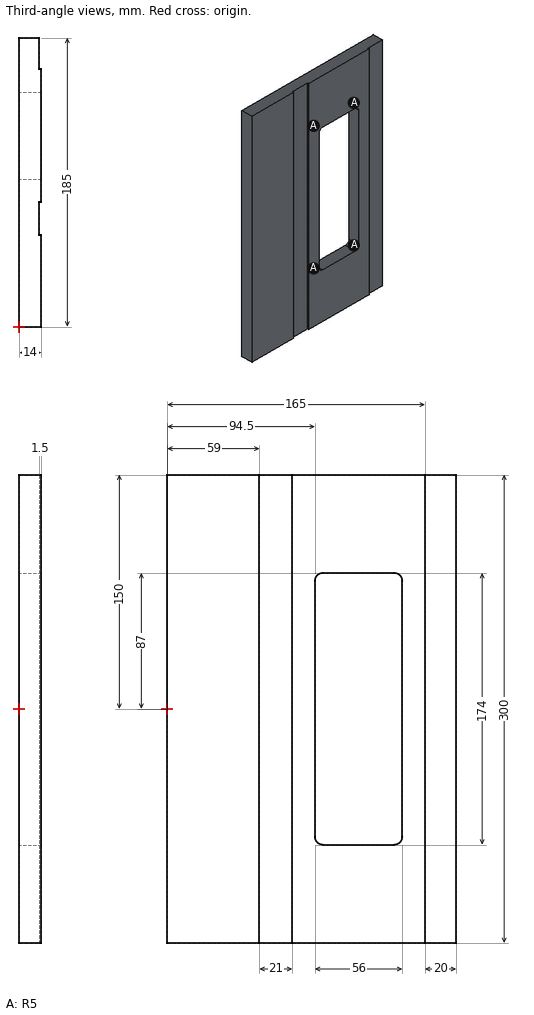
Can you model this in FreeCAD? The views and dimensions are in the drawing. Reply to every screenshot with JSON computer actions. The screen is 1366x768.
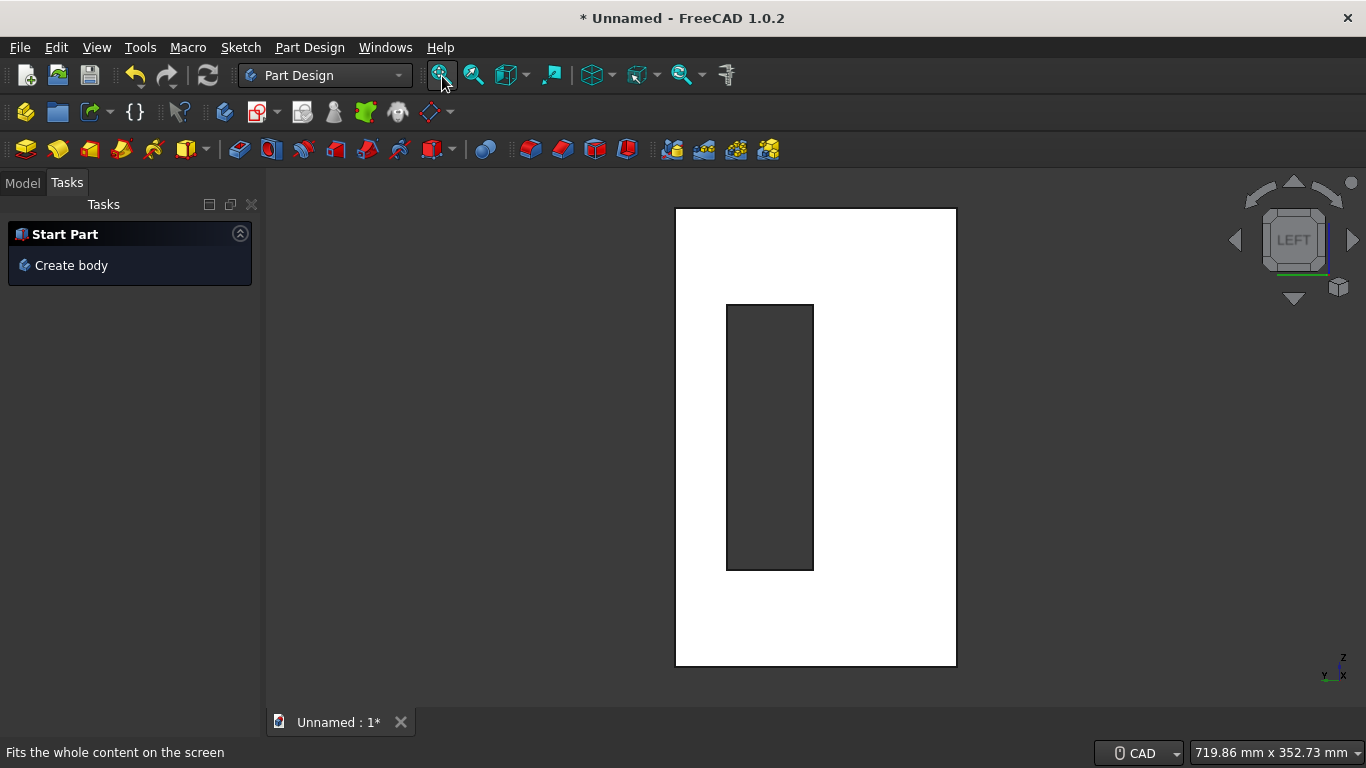
{"action": "key", "text": "0"}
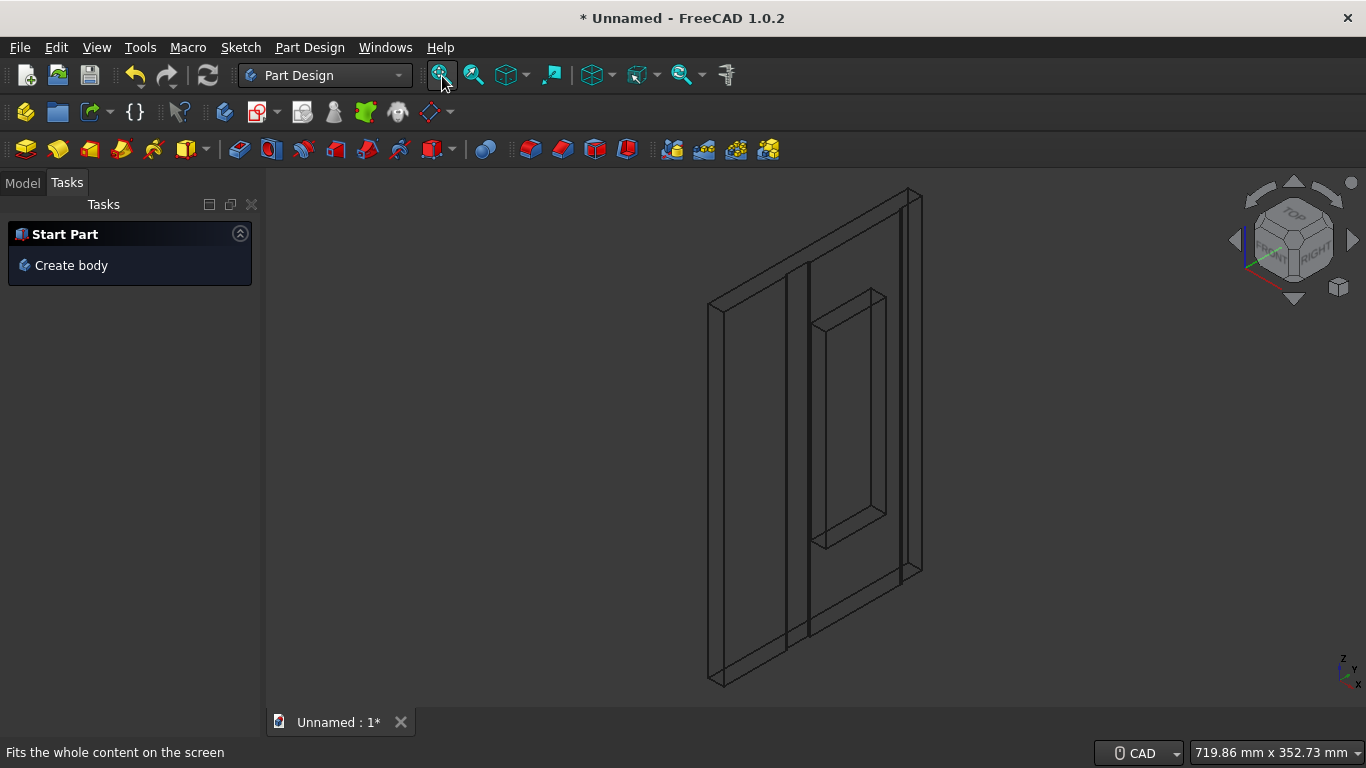
{"action": "left_click", "coordinate": [879, 509]}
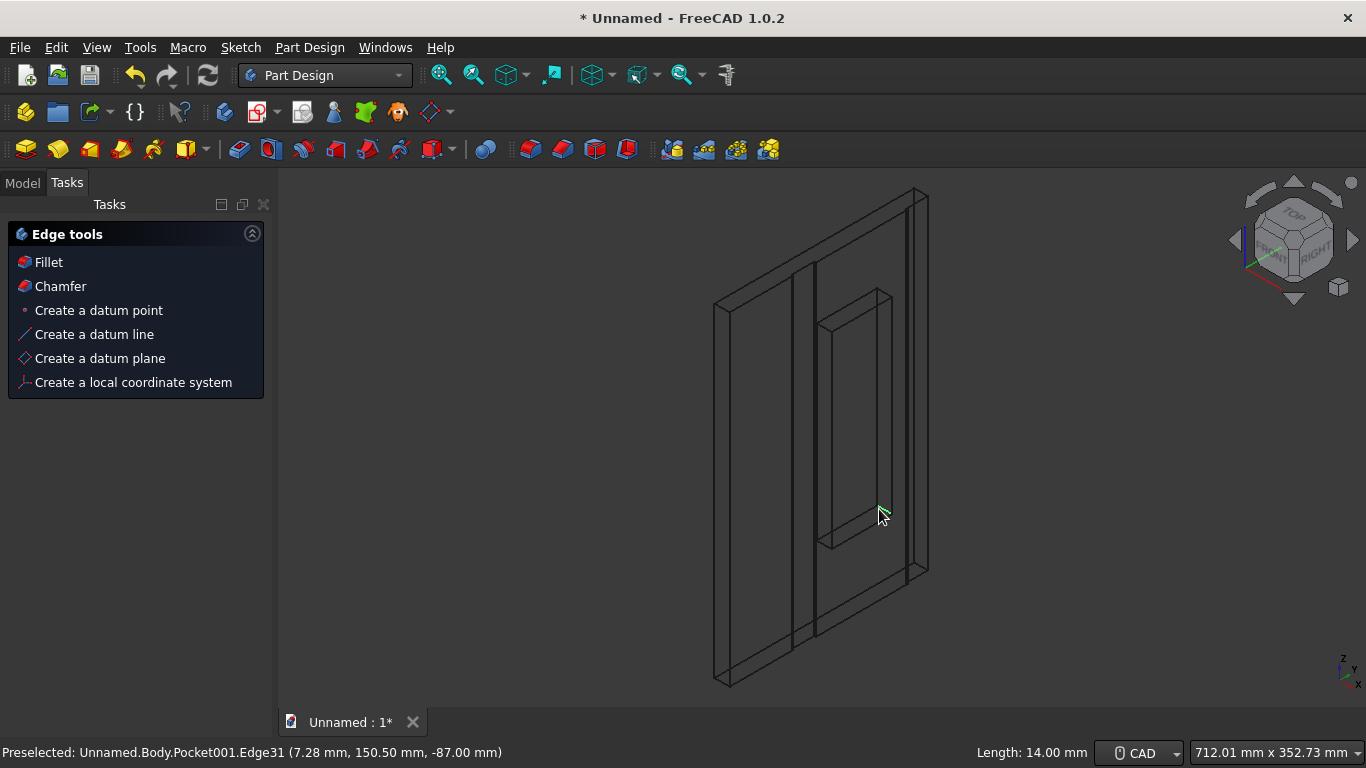
{"action": "left_click", "coordinate": [824, 544], "text": "ctrl"}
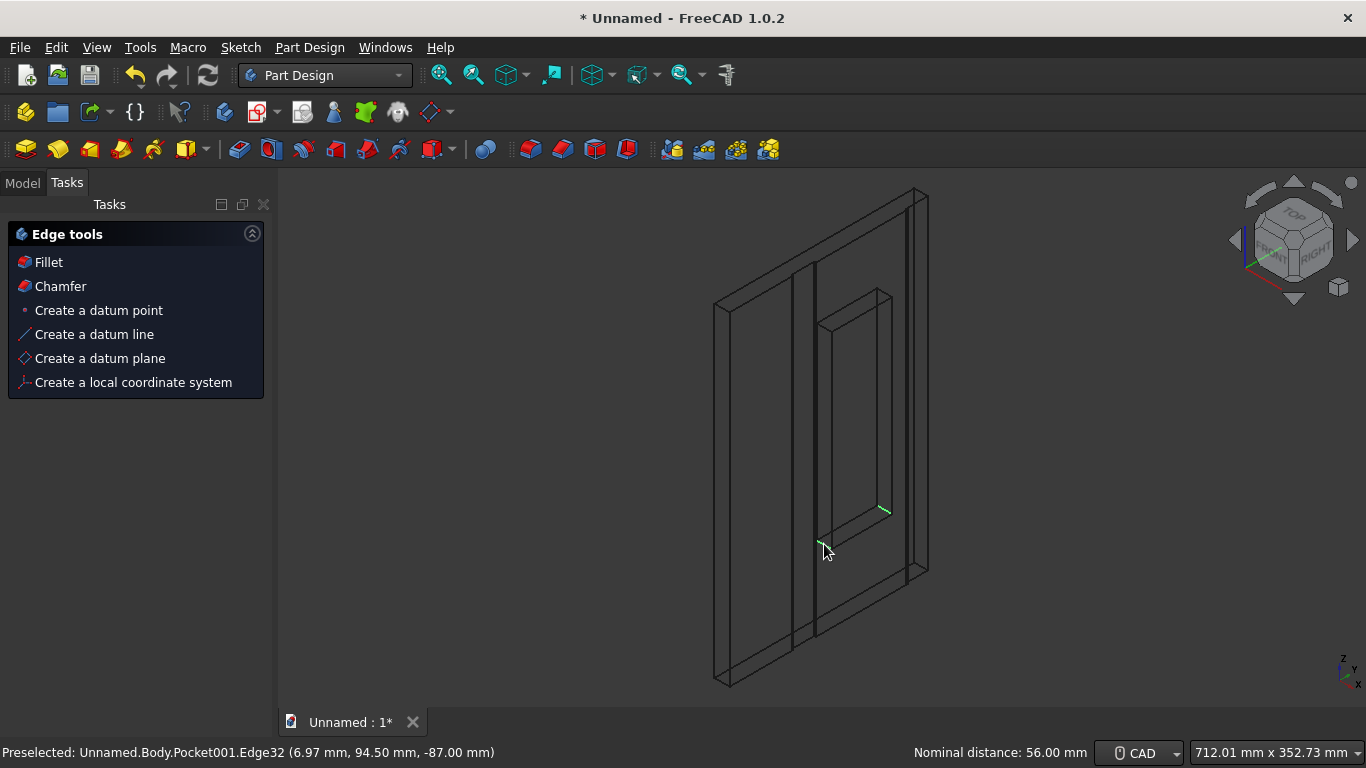
{"action": "left_click", "coordinate": [824, 327], "text": "ctrl"}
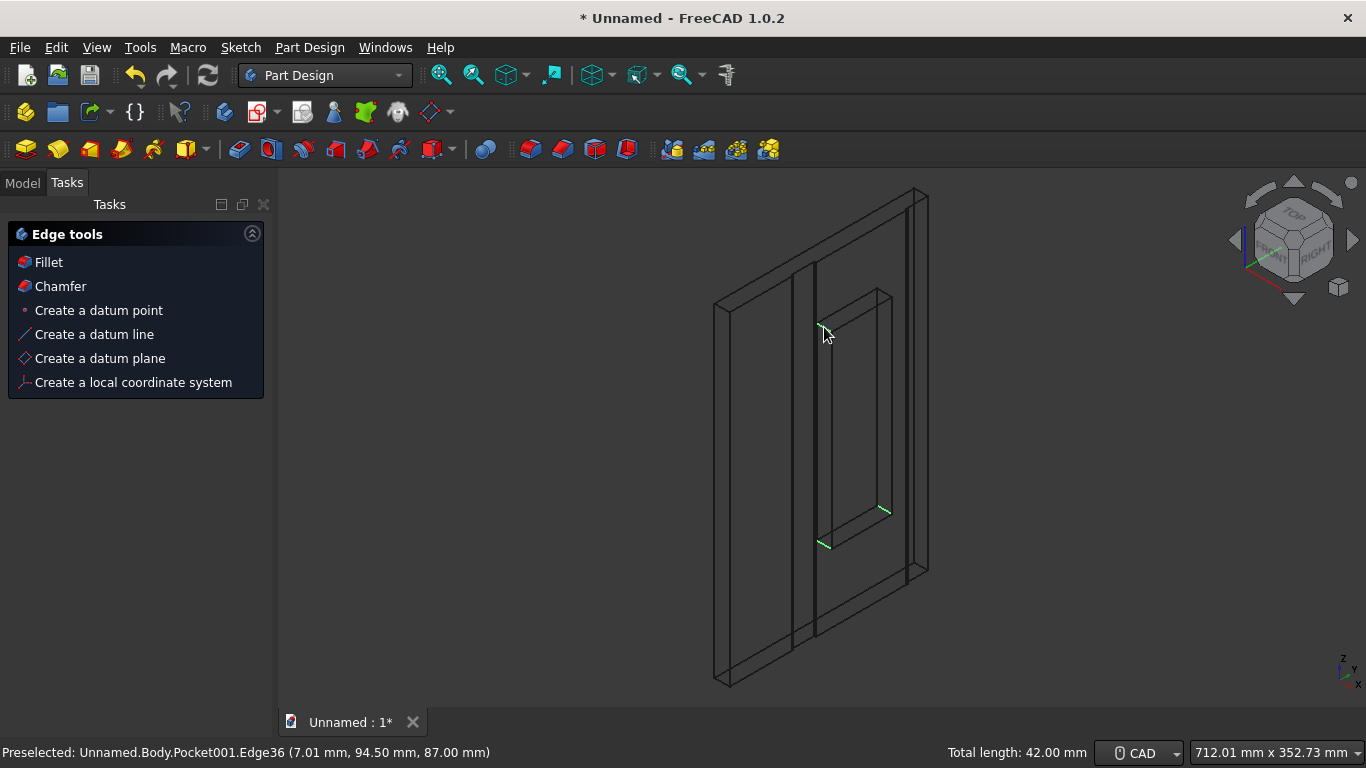
{"action": "left_click", "coordinate": [885, 292], "text": "ctrl"}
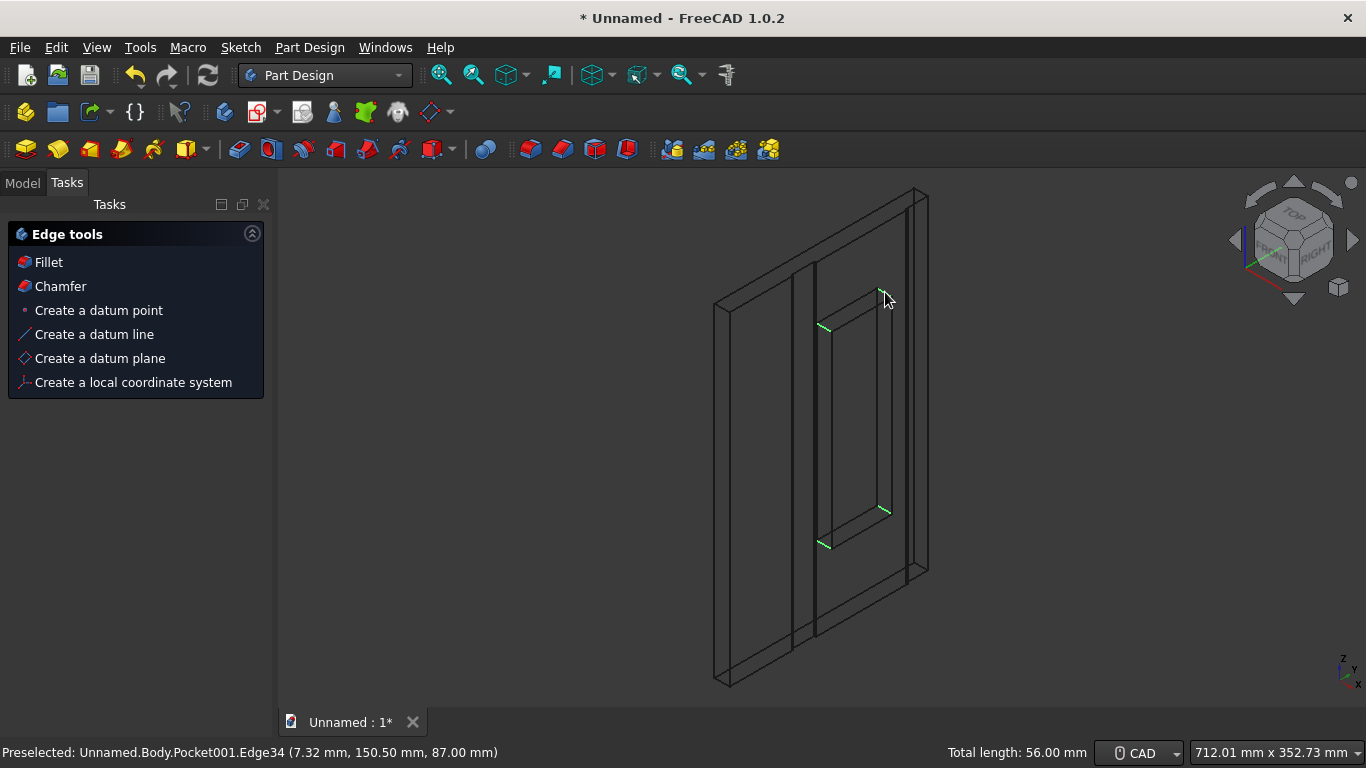
{"action": "key", "text": "v 1"}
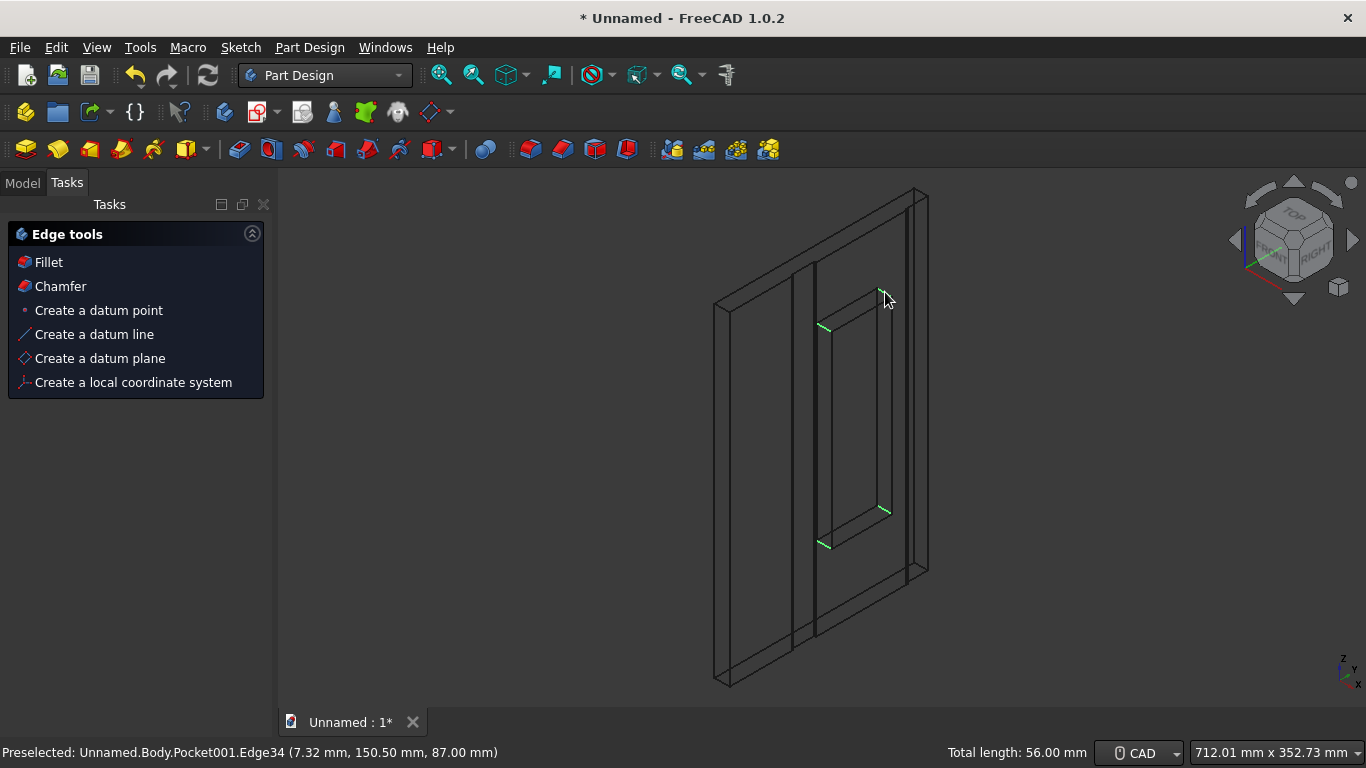
{"action": "left_click", "coordinate": [532, 150]}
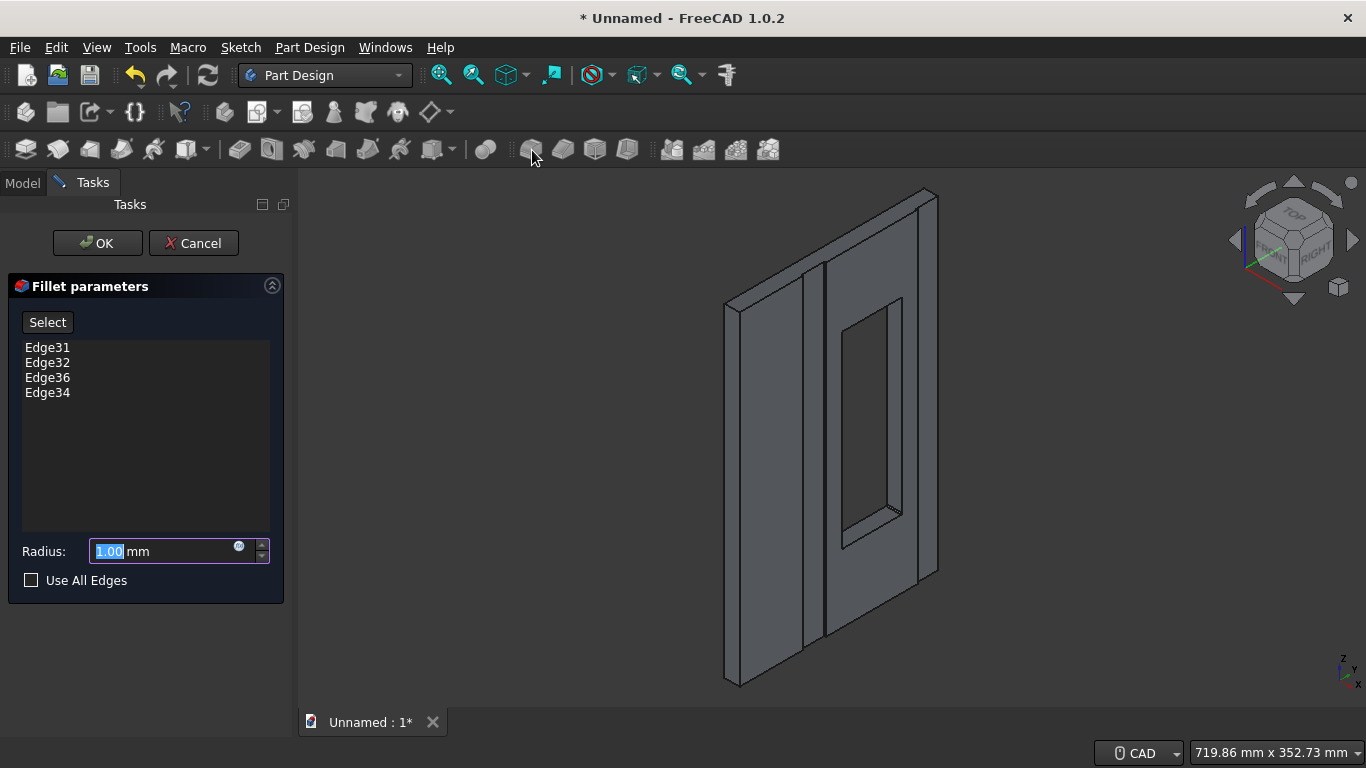
{"action": "type", "text": "5"}
{"action": "key", "text": "Tab"}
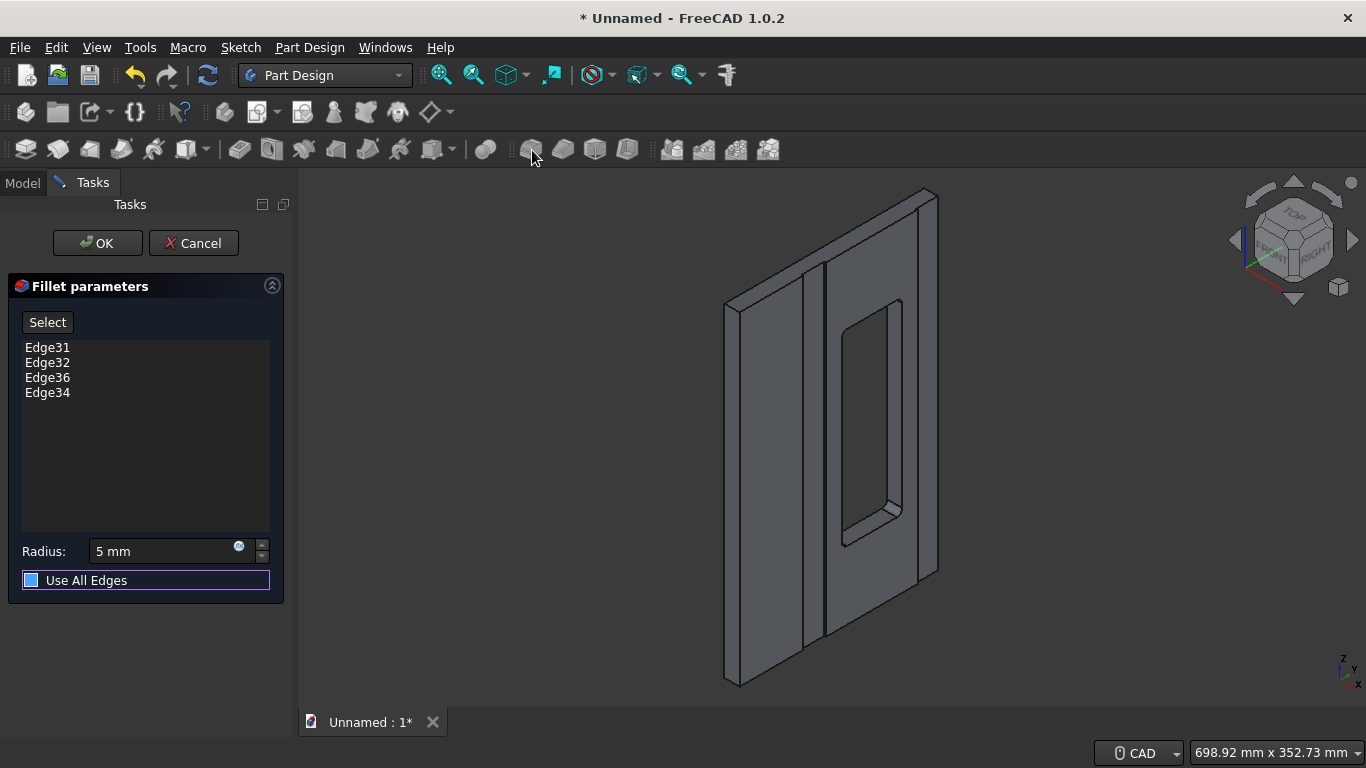
{"action": "left_click", "coordinate": [98, 243]}